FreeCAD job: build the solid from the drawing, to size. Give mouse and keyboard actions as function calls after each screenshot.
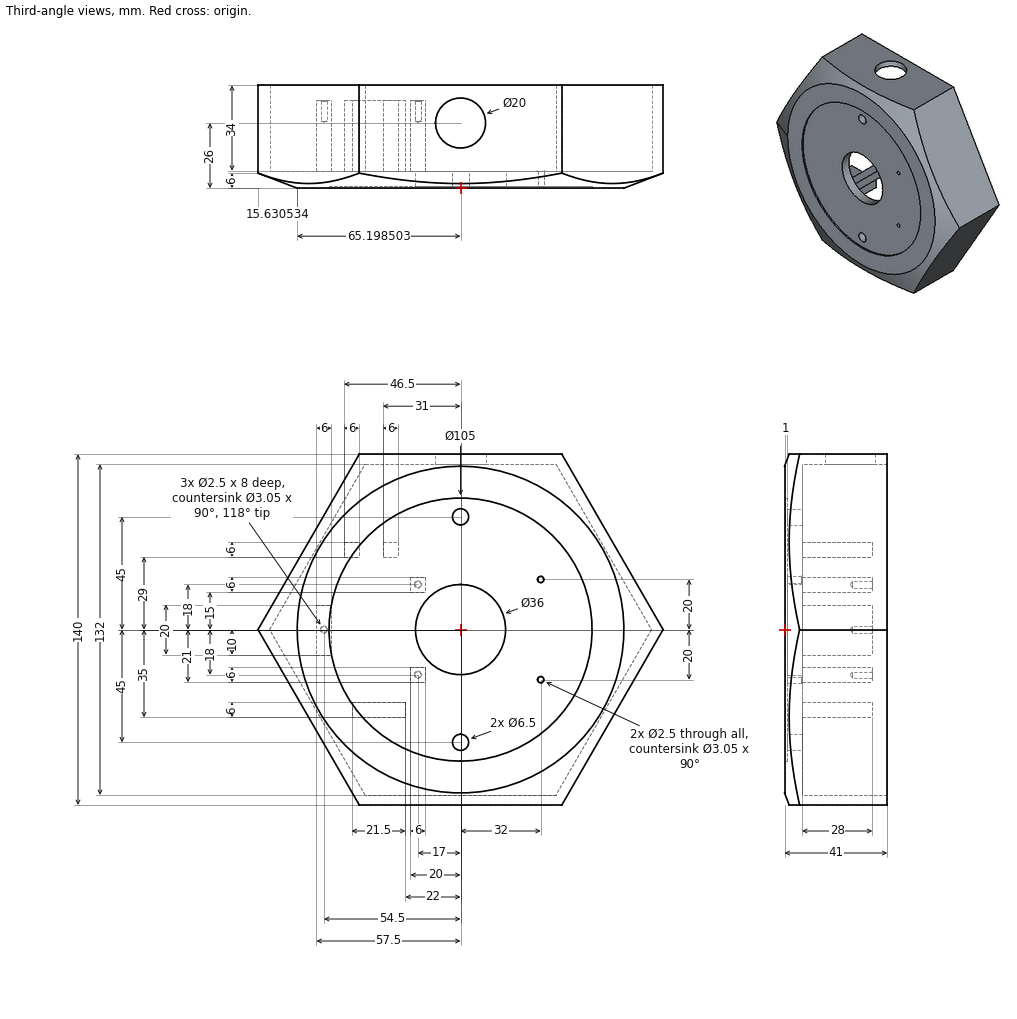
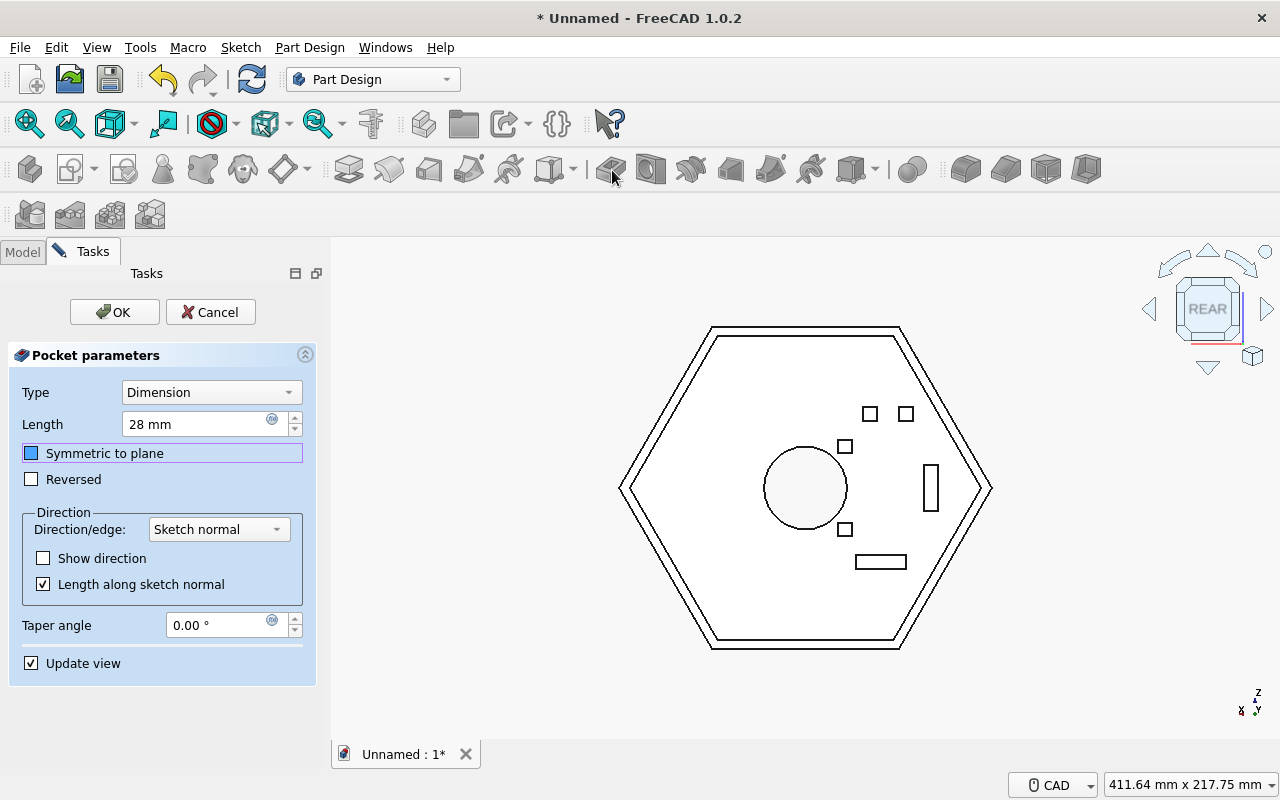
click(115, 312)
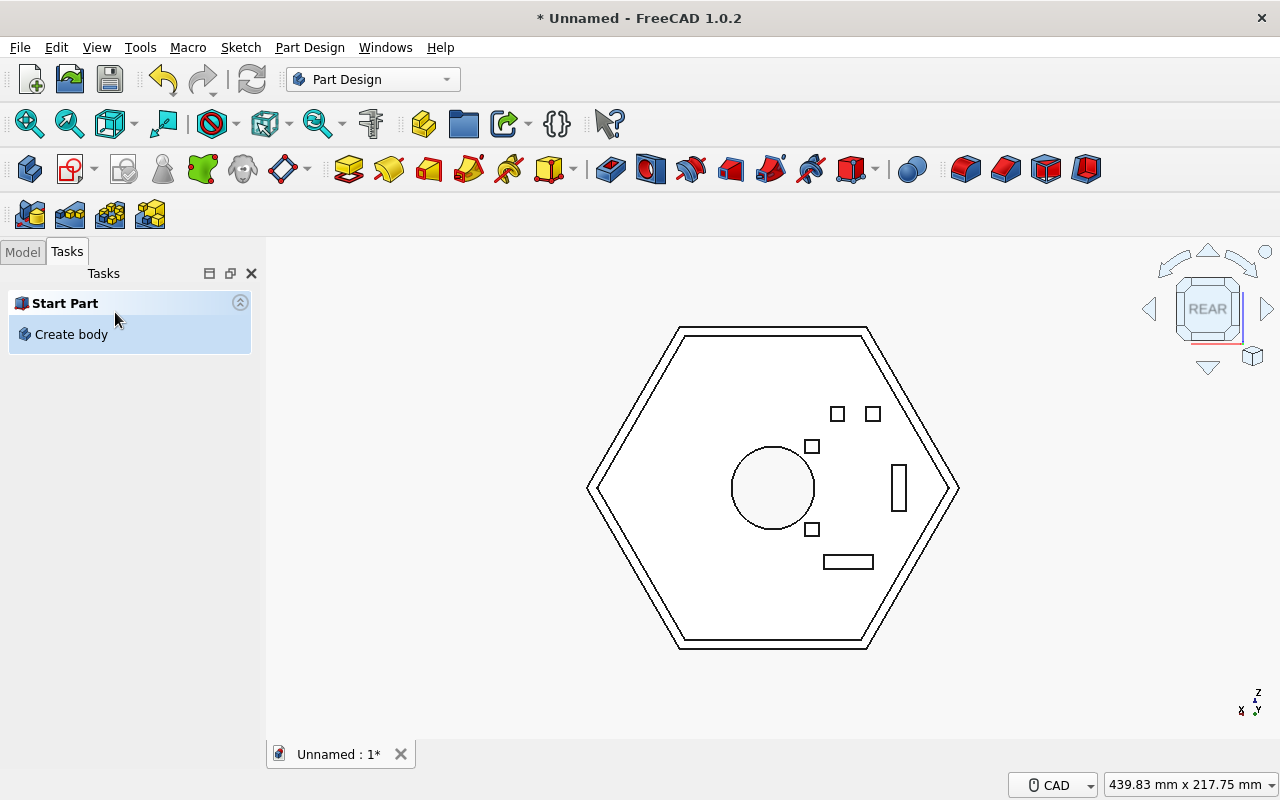
click(723, 400)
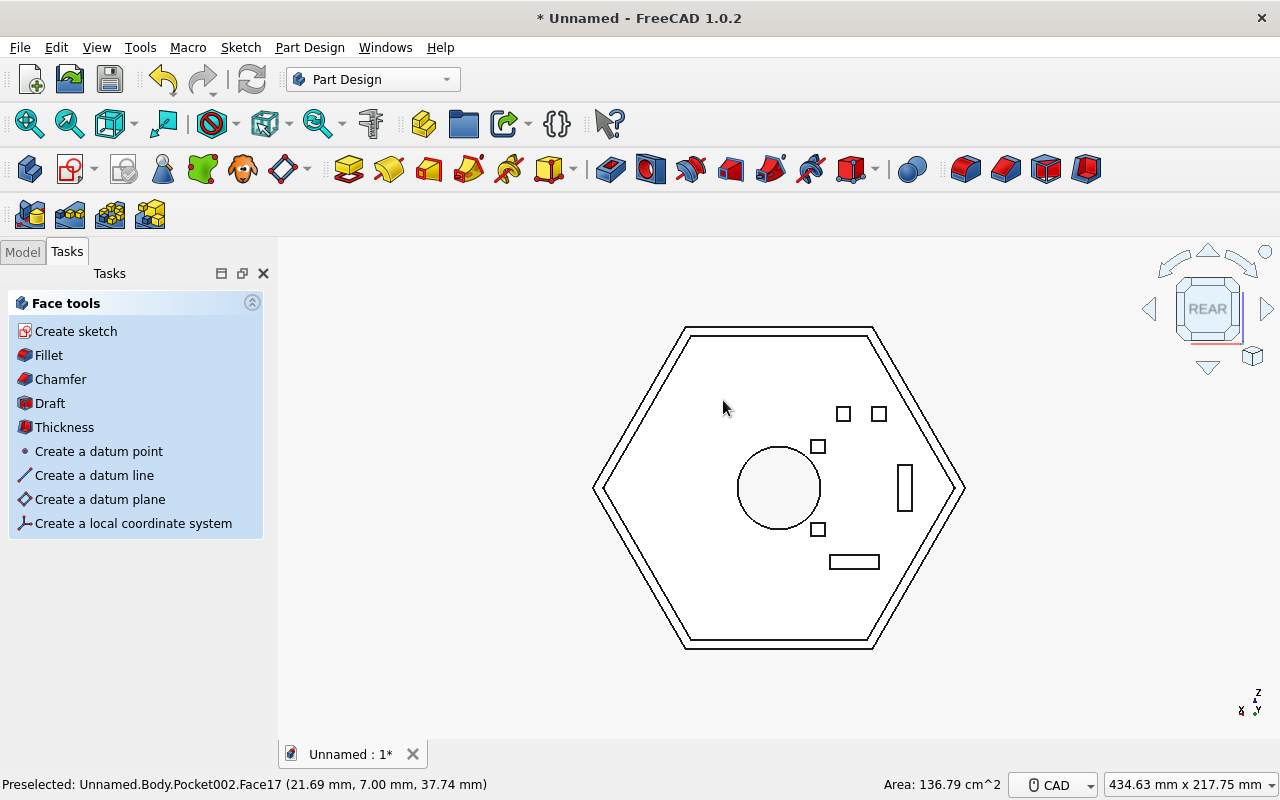
click(70, 170)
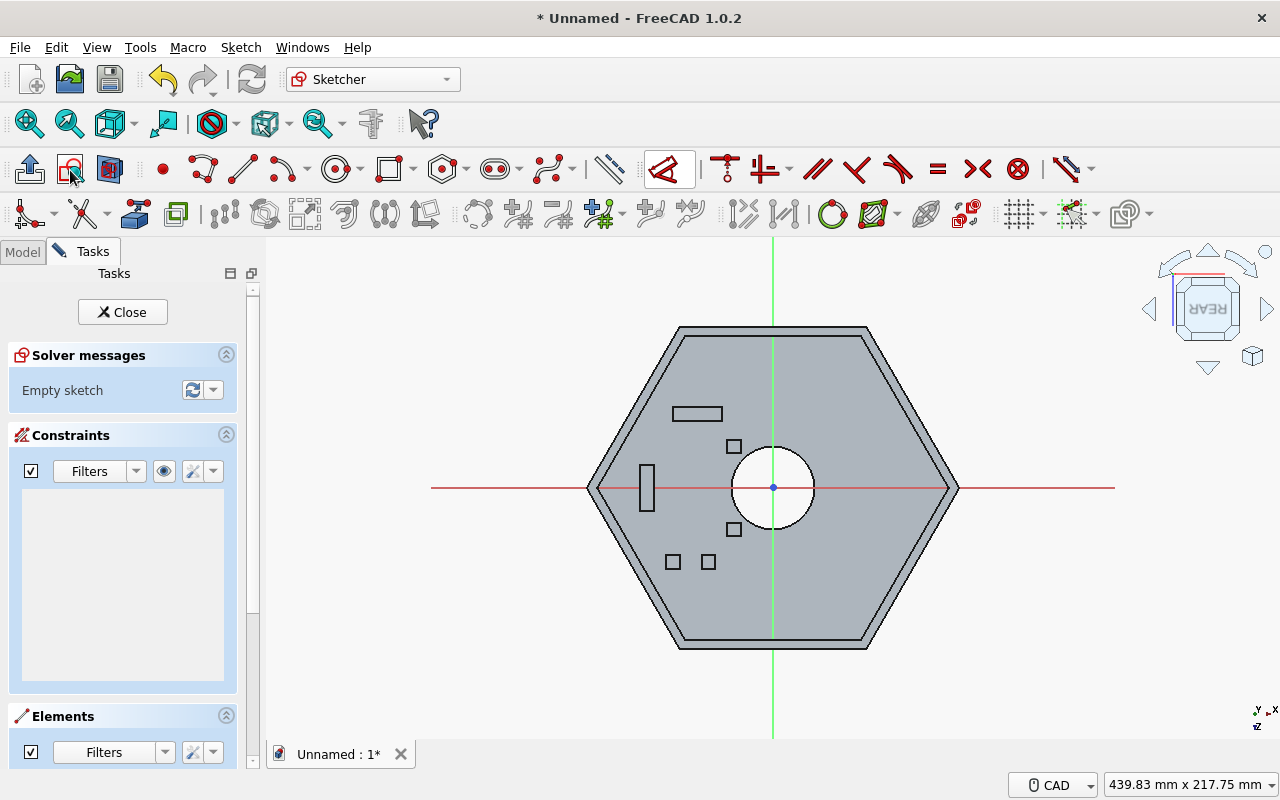
click(110, 170)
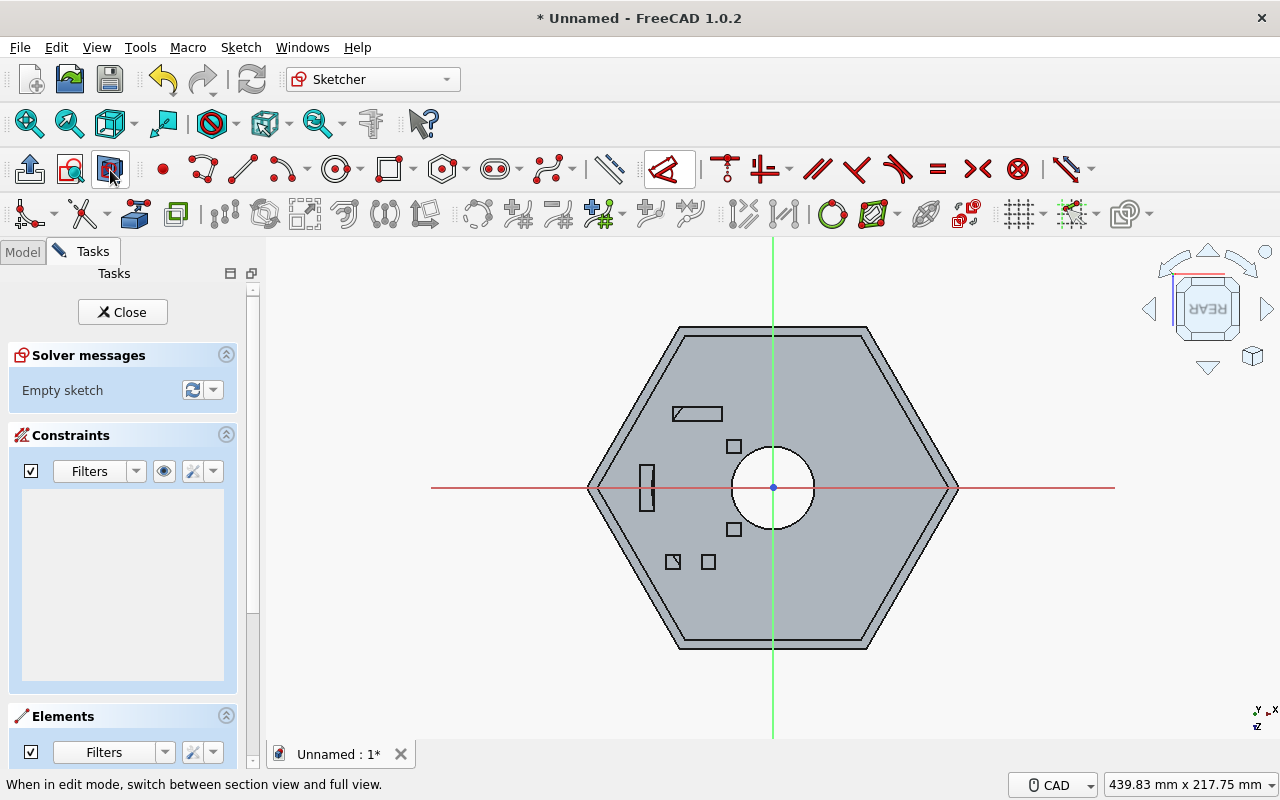
scroll(912, 488, up, 2)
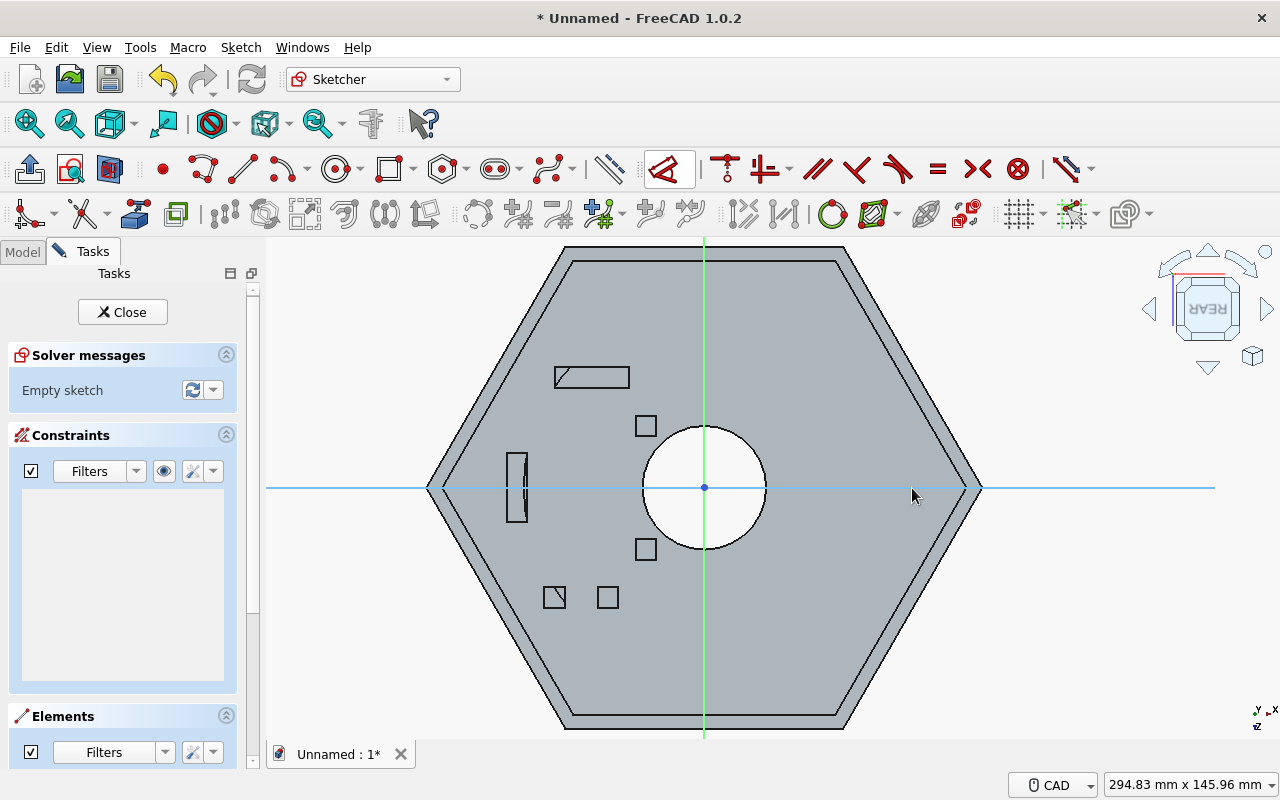
key(g)
key(c)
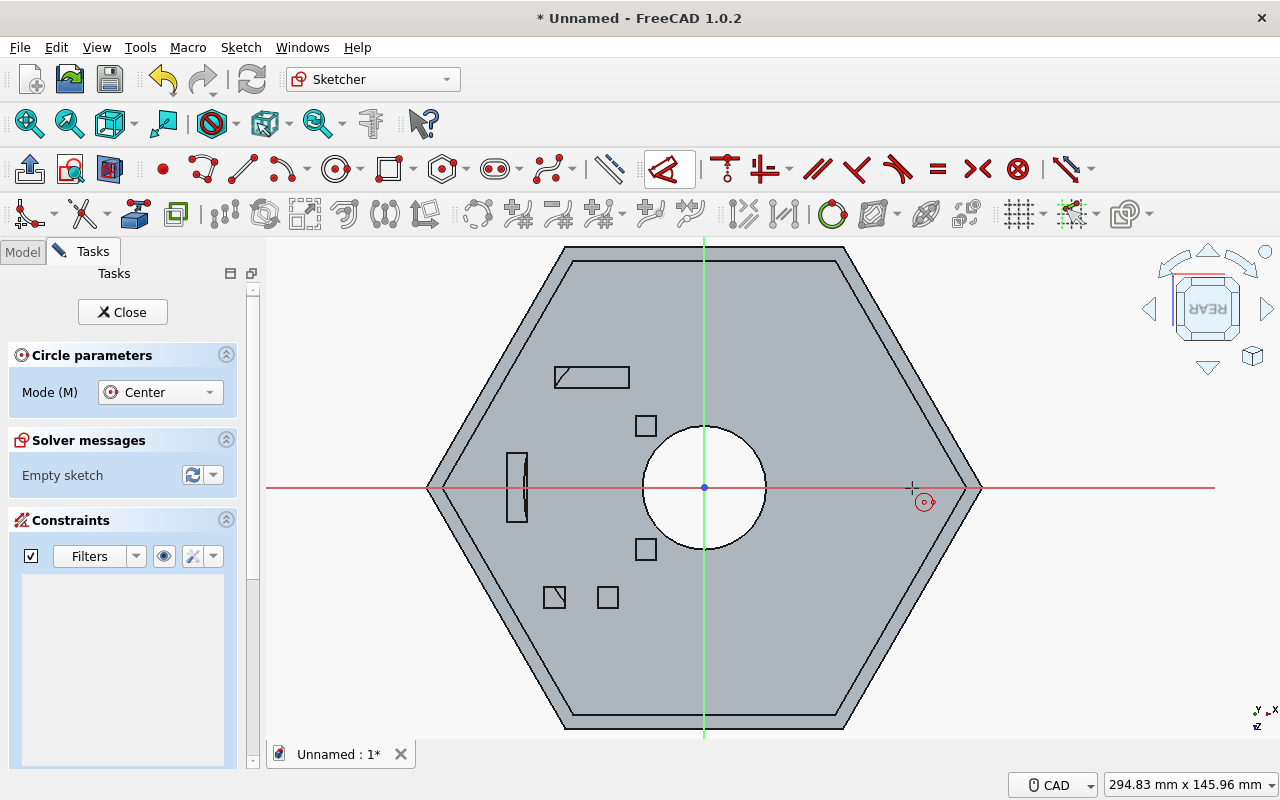
scroll(704, 333, up, 4)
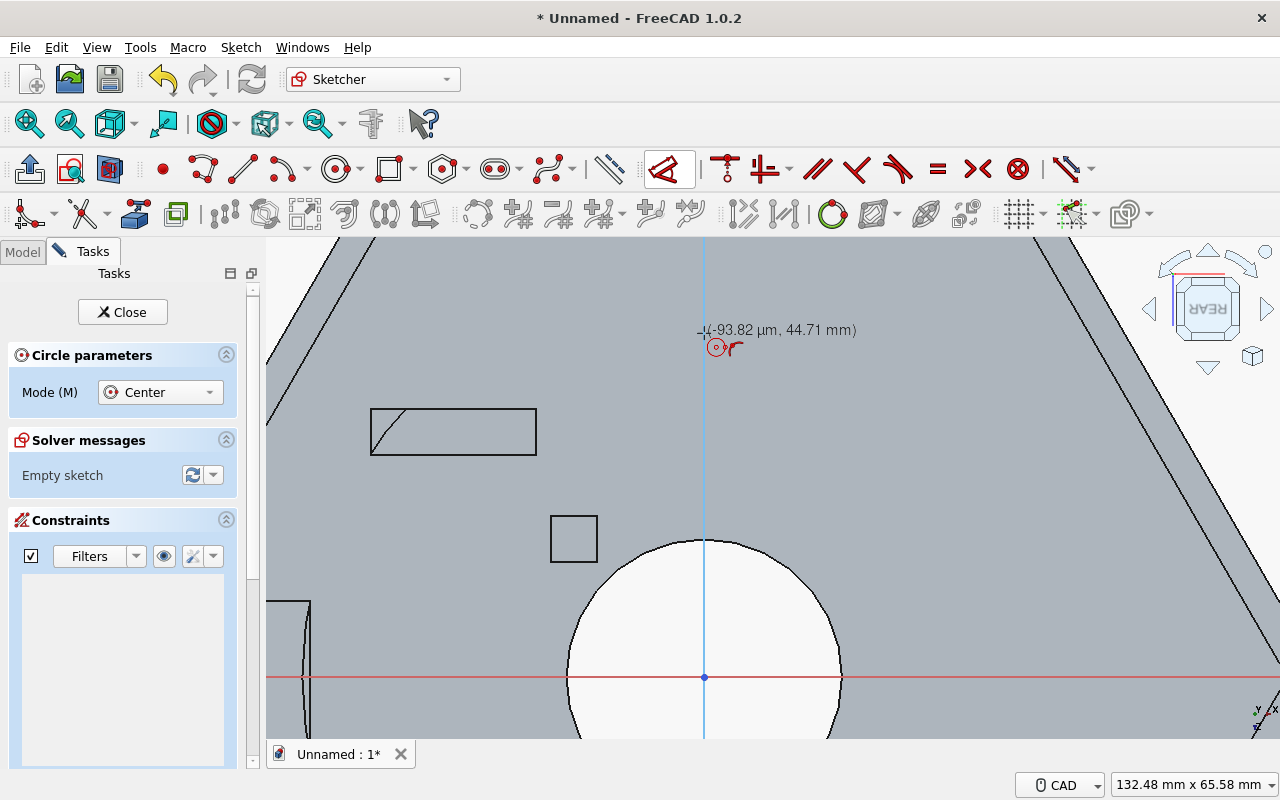
click(704, 333)
move(722, 315)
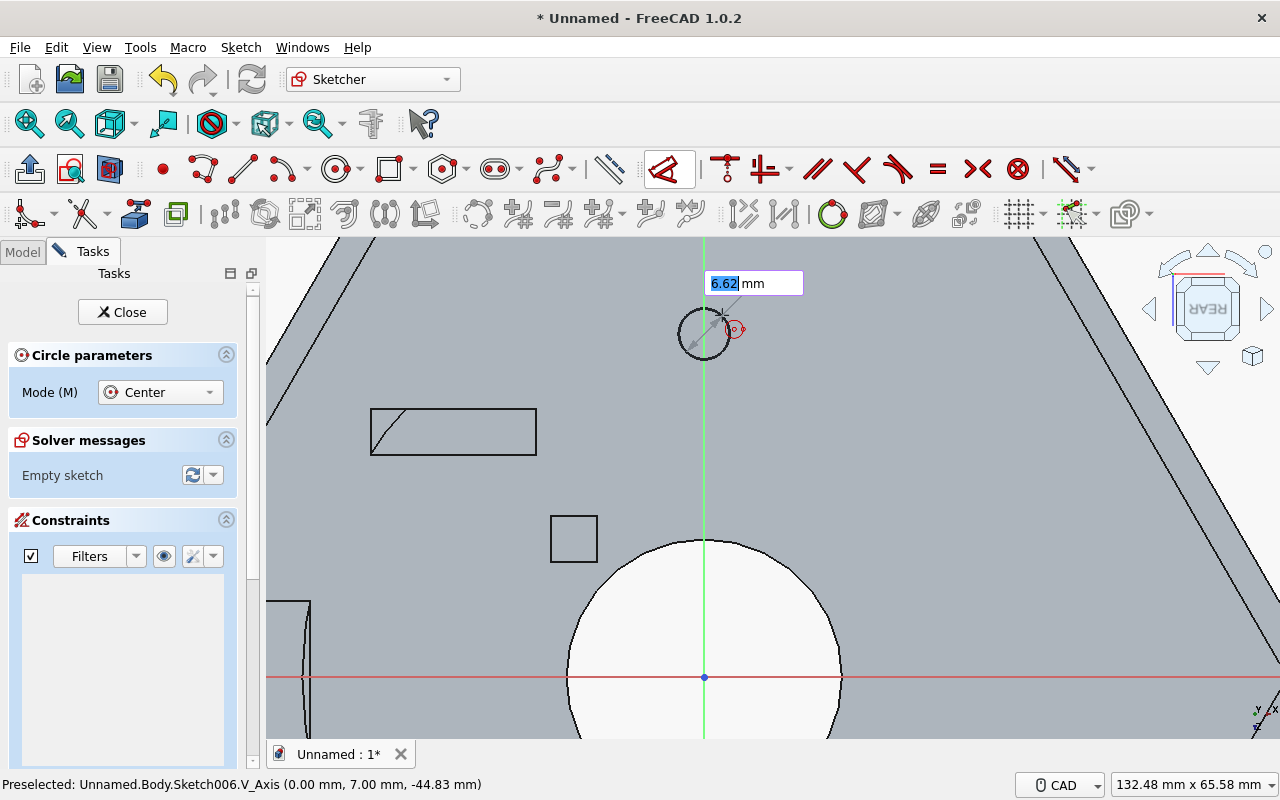
text(6.5)
key(Return)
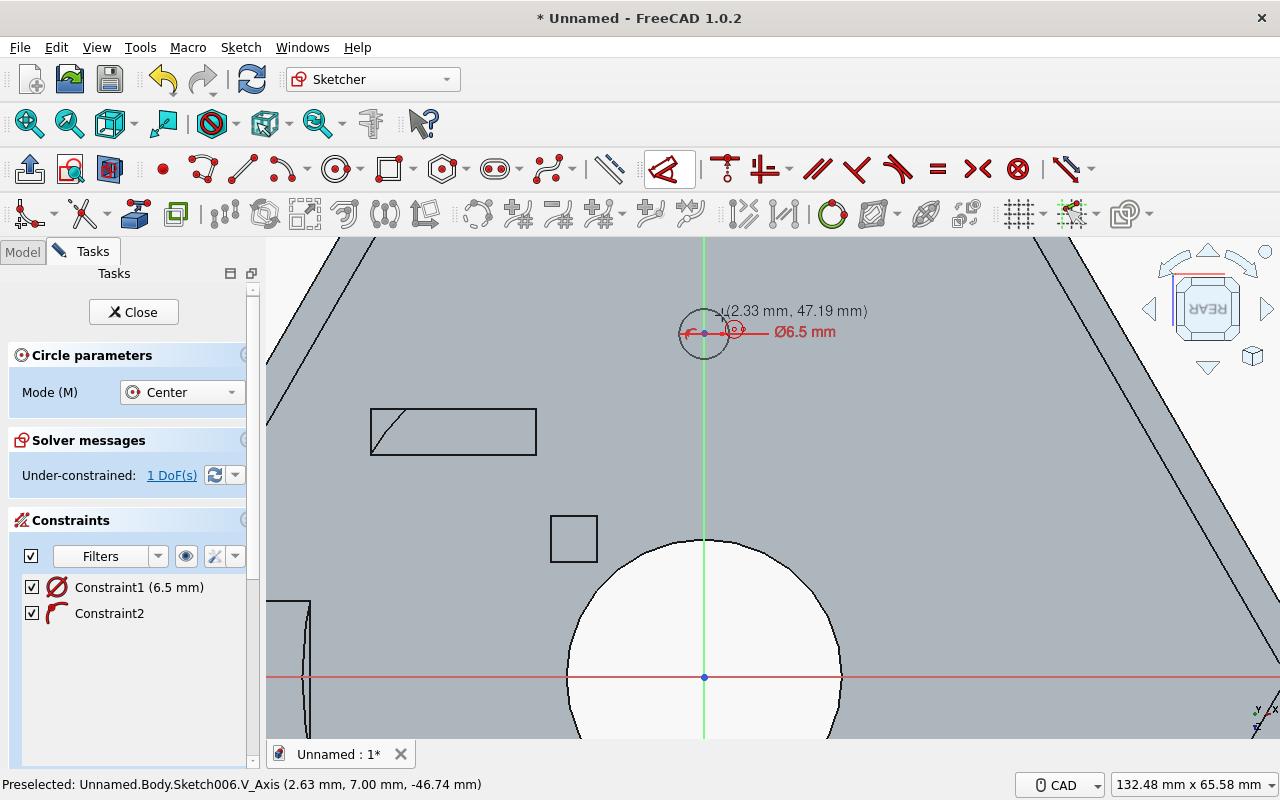
scroll(705, 334, down, 4)